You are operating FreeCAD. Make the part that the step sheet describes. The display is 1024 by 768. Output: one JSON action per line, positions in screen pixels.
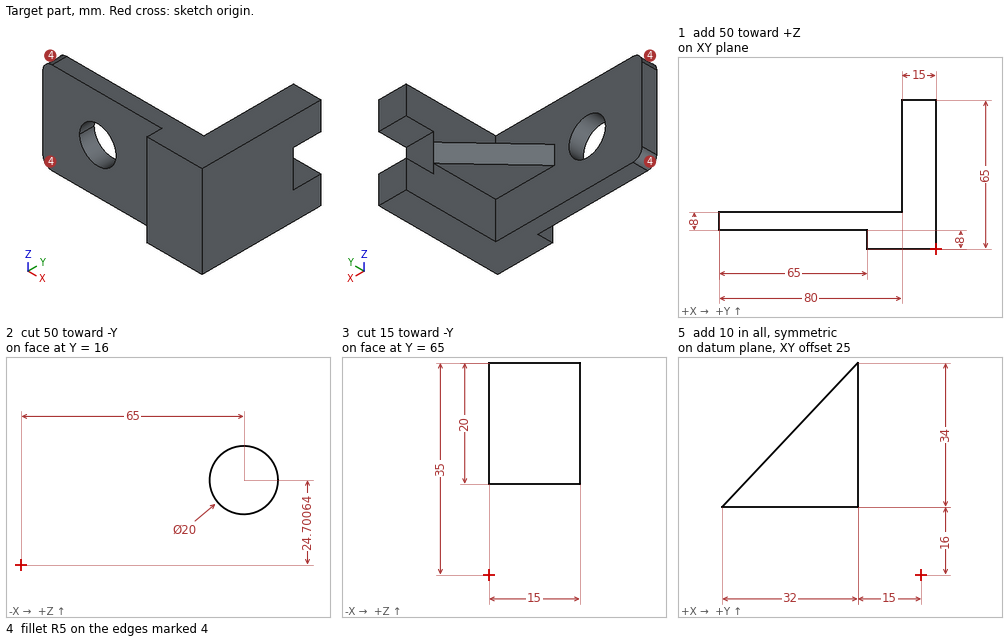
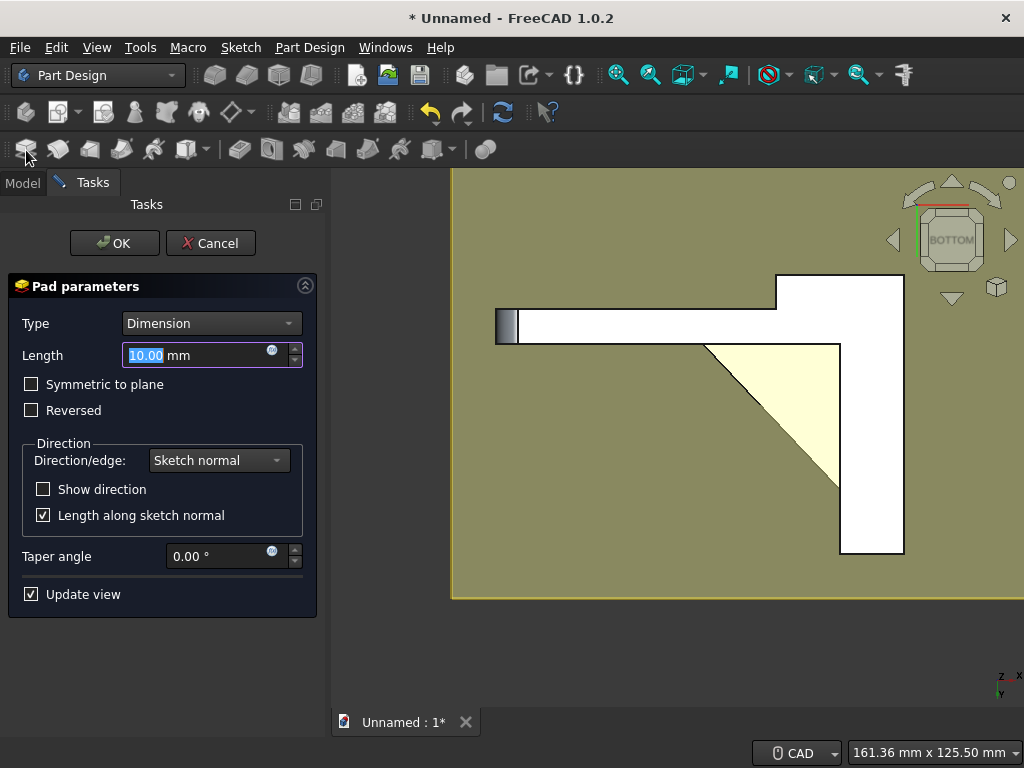
{"action": "type", "text": "10"}
{"action": "key", "text": "Tab"}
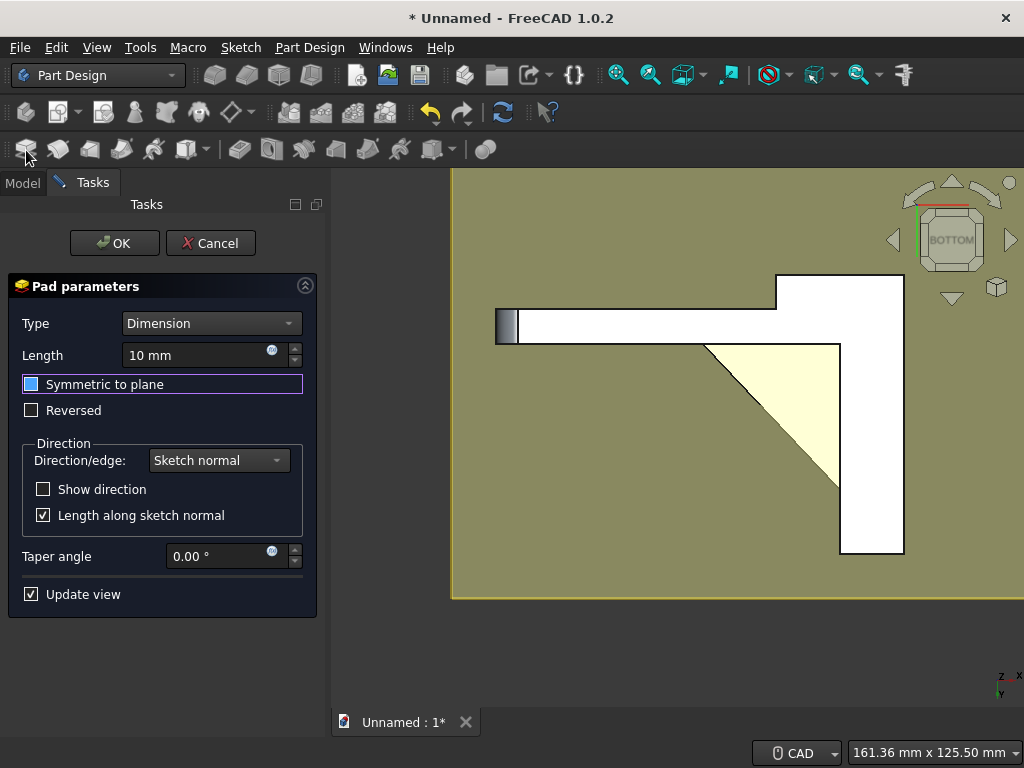
{"action": "left_click", "coordinate": [30, 384]}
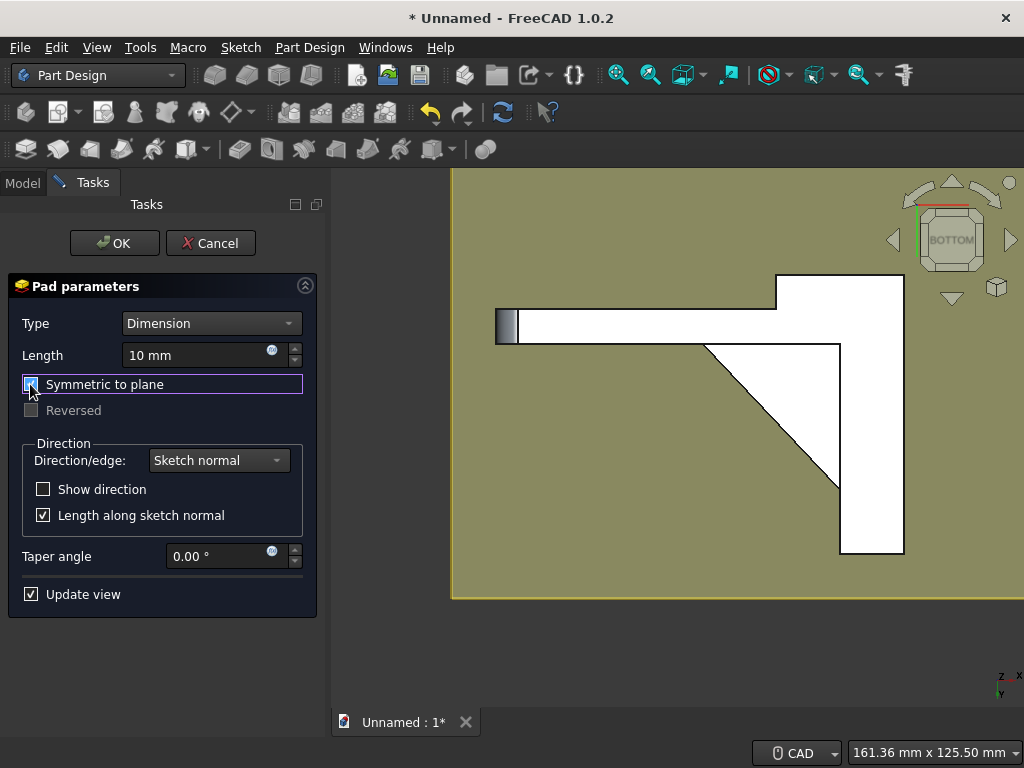
{"action": "left_click", "coordinate": [115, 243]}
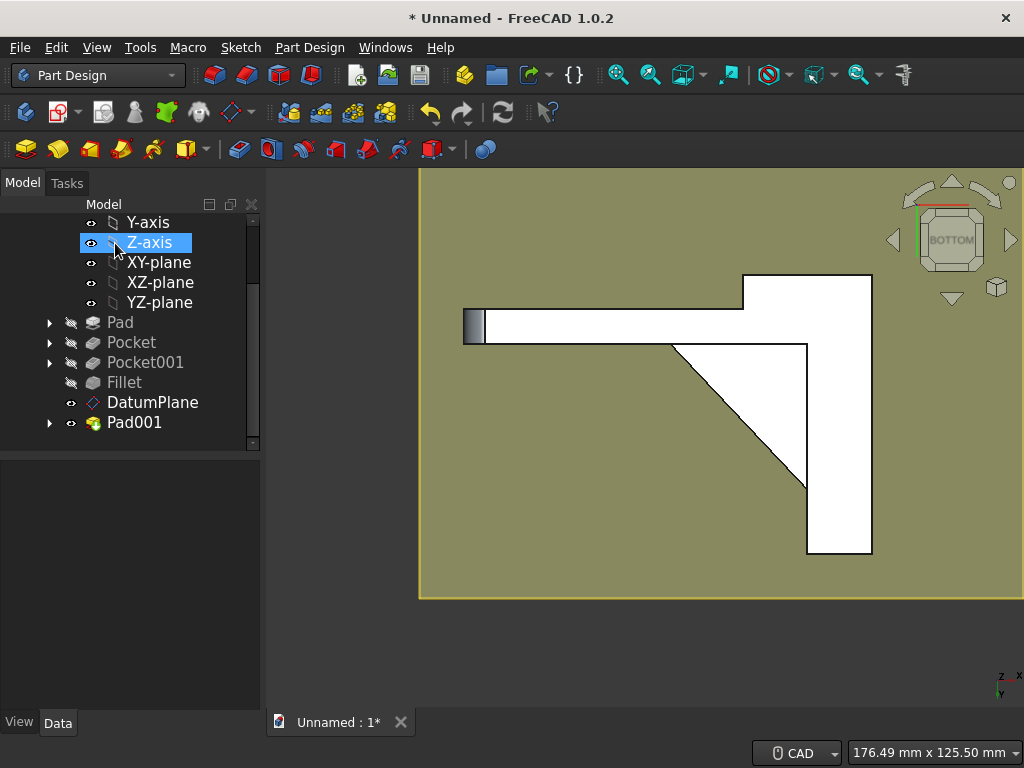
{"action": "left_click", "coordinate": [116, 403]}
{"action": "key", "text": "space"}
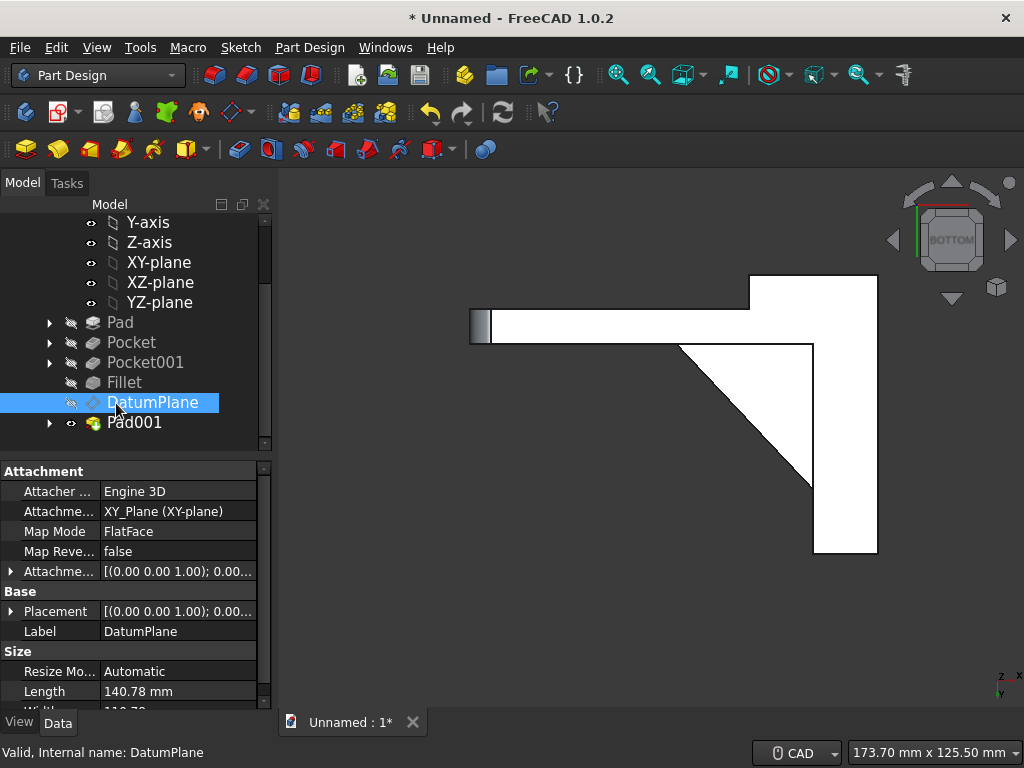
{"action": "key", "text": "0"}